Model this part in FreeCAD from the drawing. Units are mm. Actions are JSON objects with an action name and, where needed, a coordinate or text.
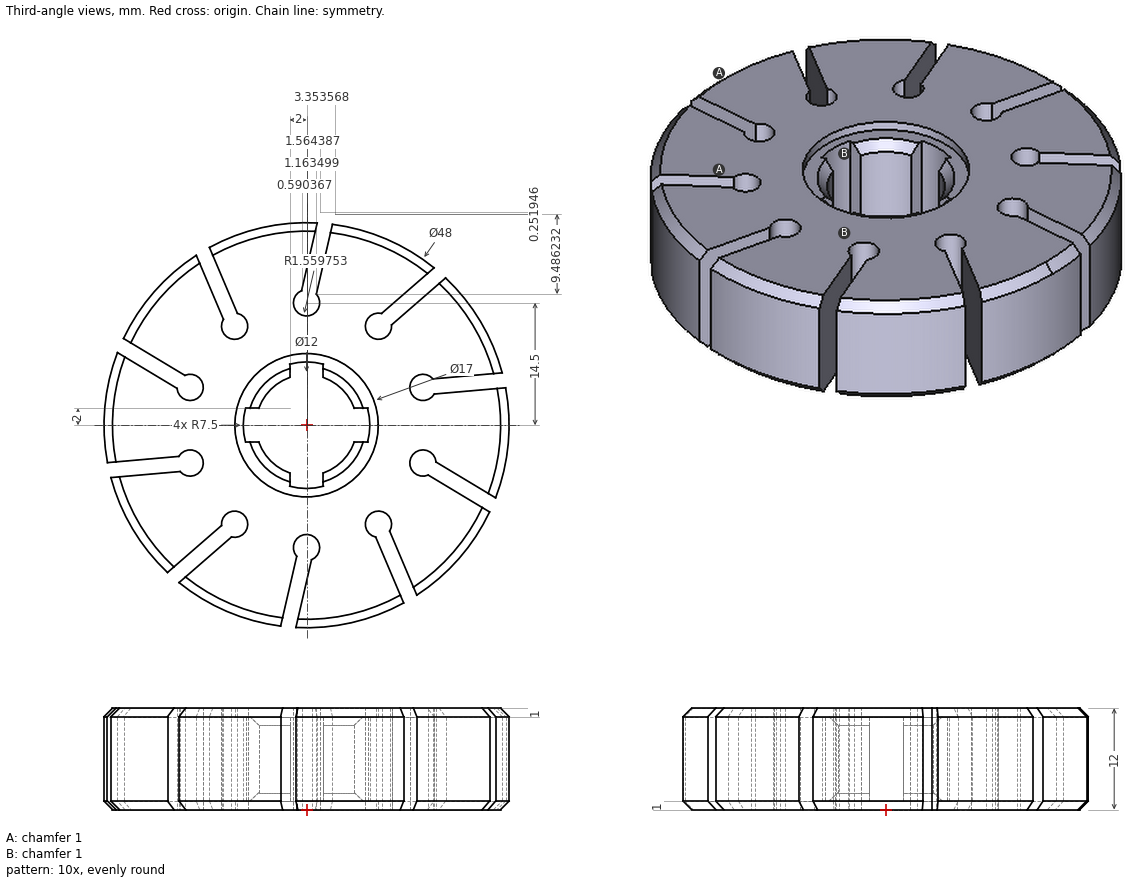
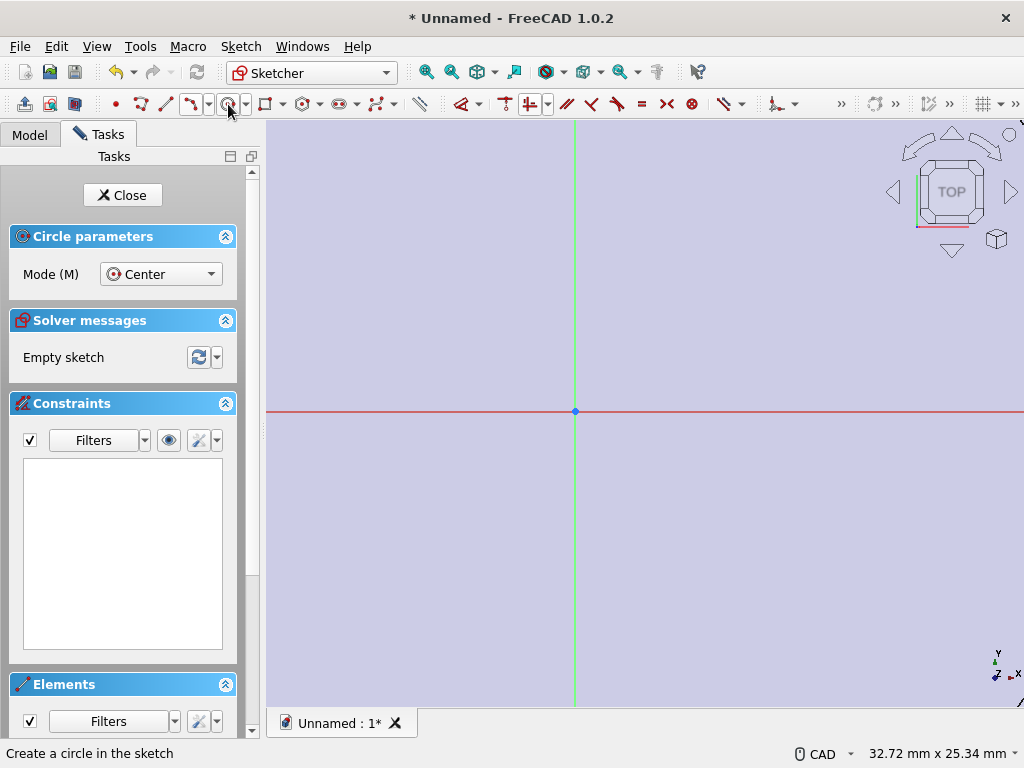
{"action": "left_click", "coordinate": [575, 412]}
{"action": "mouse_move", "coordinate": [715, 273]}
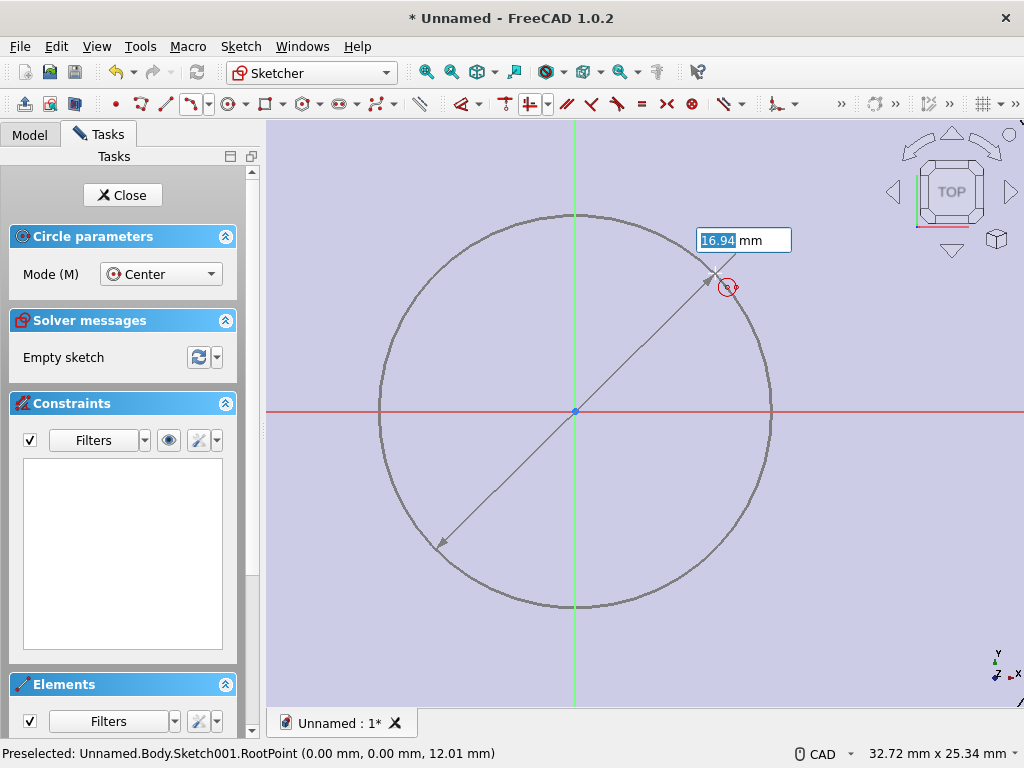
{"action": "type", "text": "17"}
{"action": "key", "text": "Return"}
{"action": "key", "text": "Escape"}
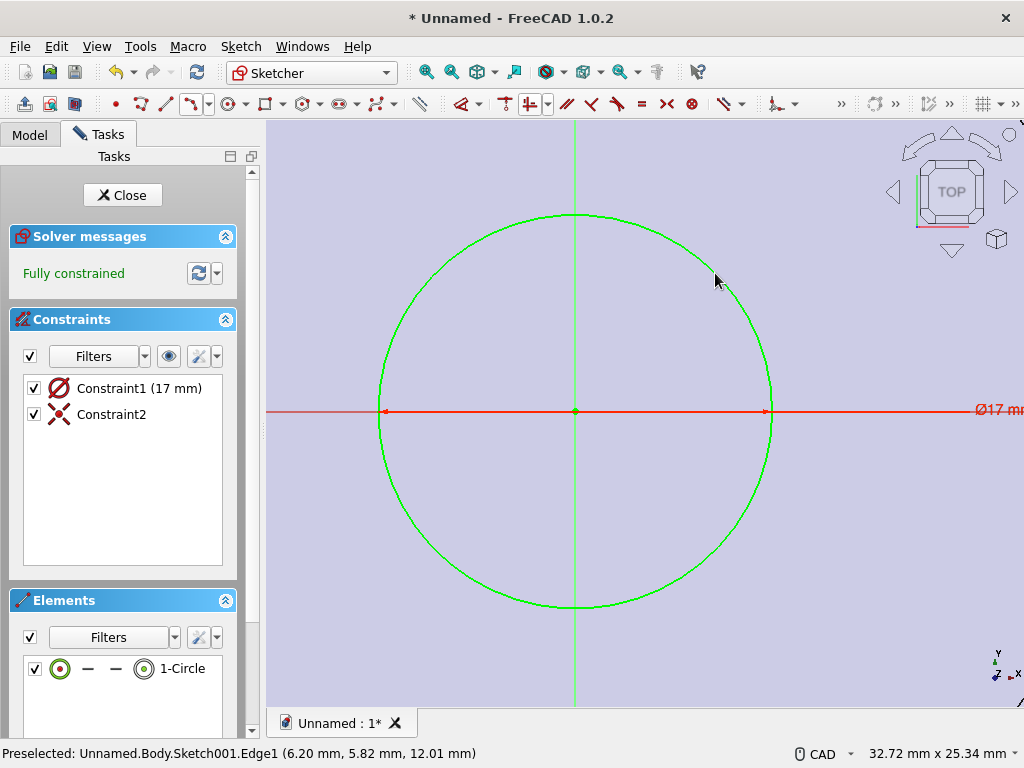
{"action": "left_click", "coordinate": [123, 195]}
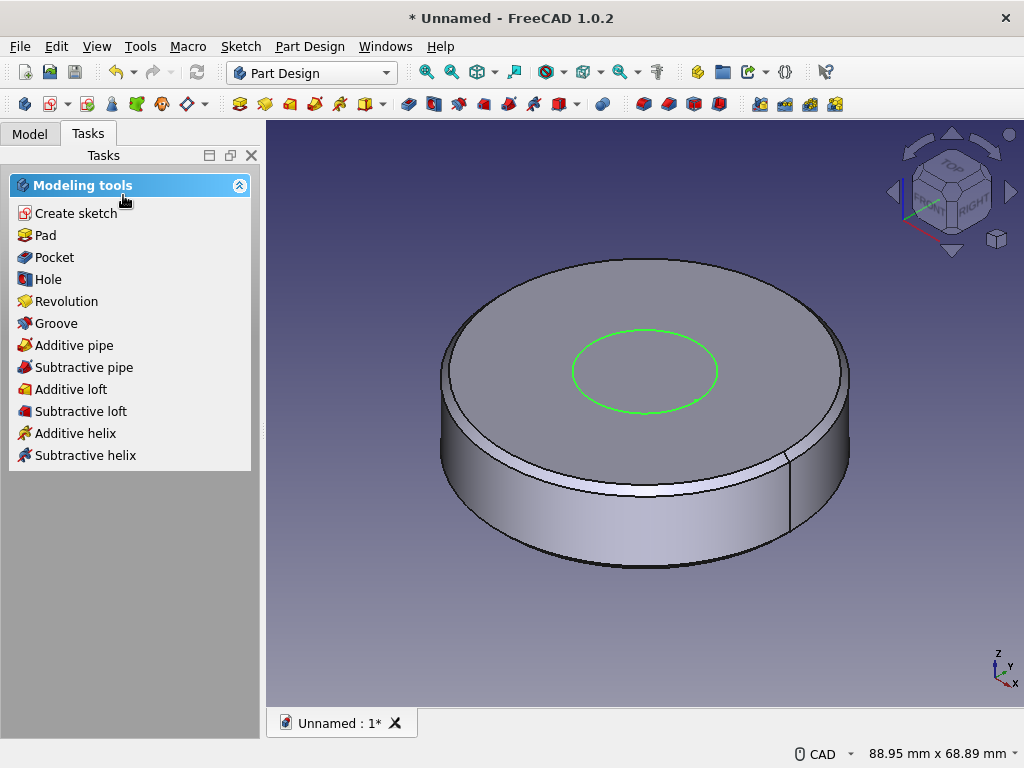
{"action": "left_click", "coordinate": [409, 104]}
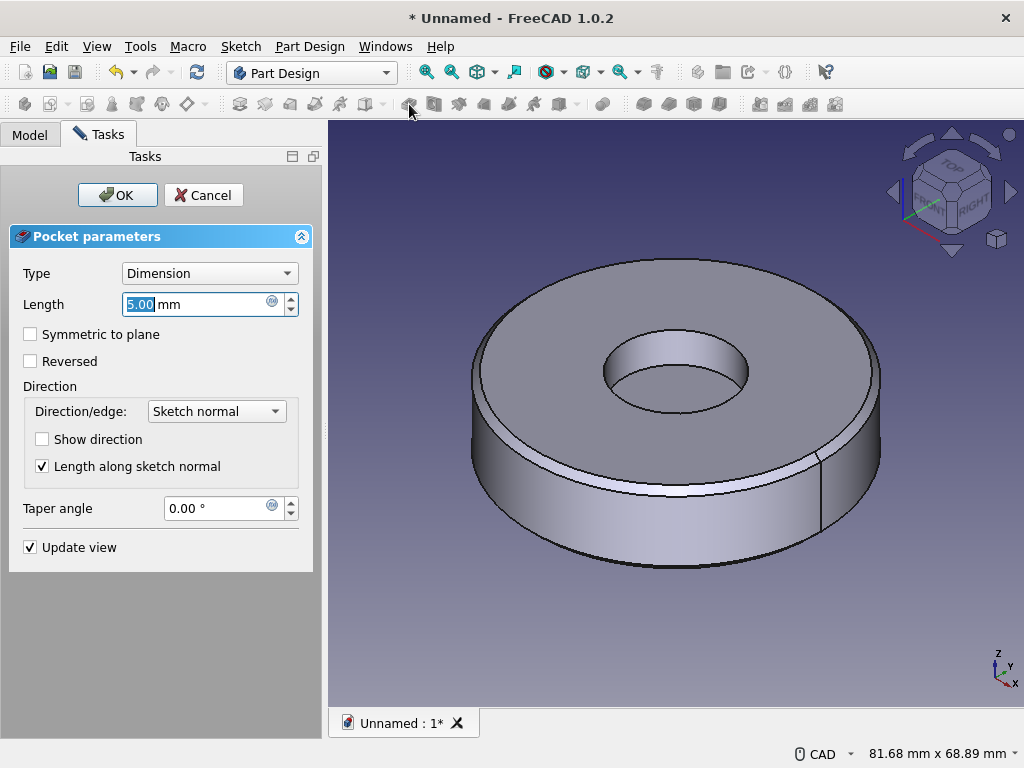
{"action": "type", "text": "1"}
{"action": "key", "text": "Tab"}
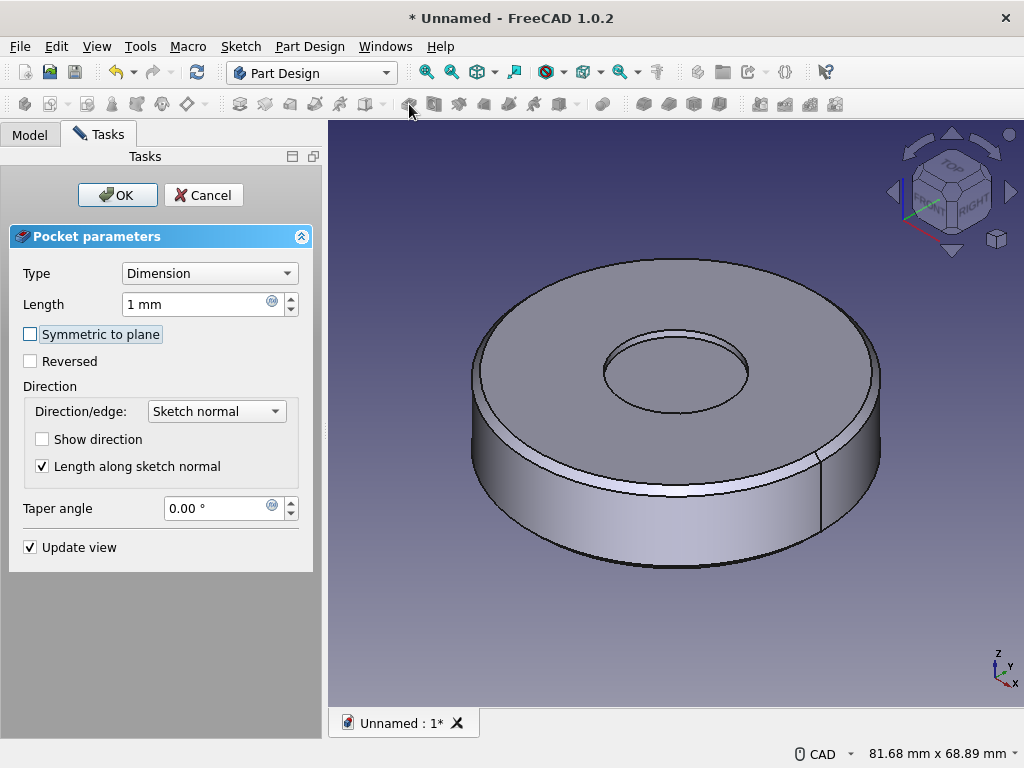
{"action": "left_click", "coordinate": [118, 195]}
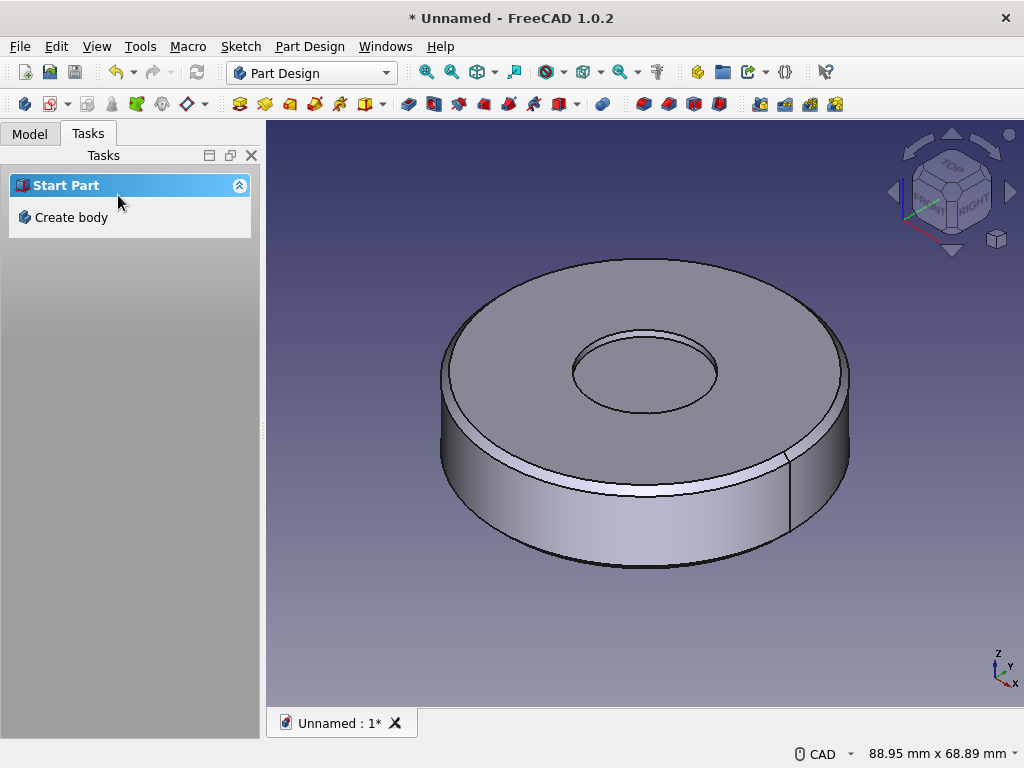
{"action": "left_click", "coordinate": [30, 134]}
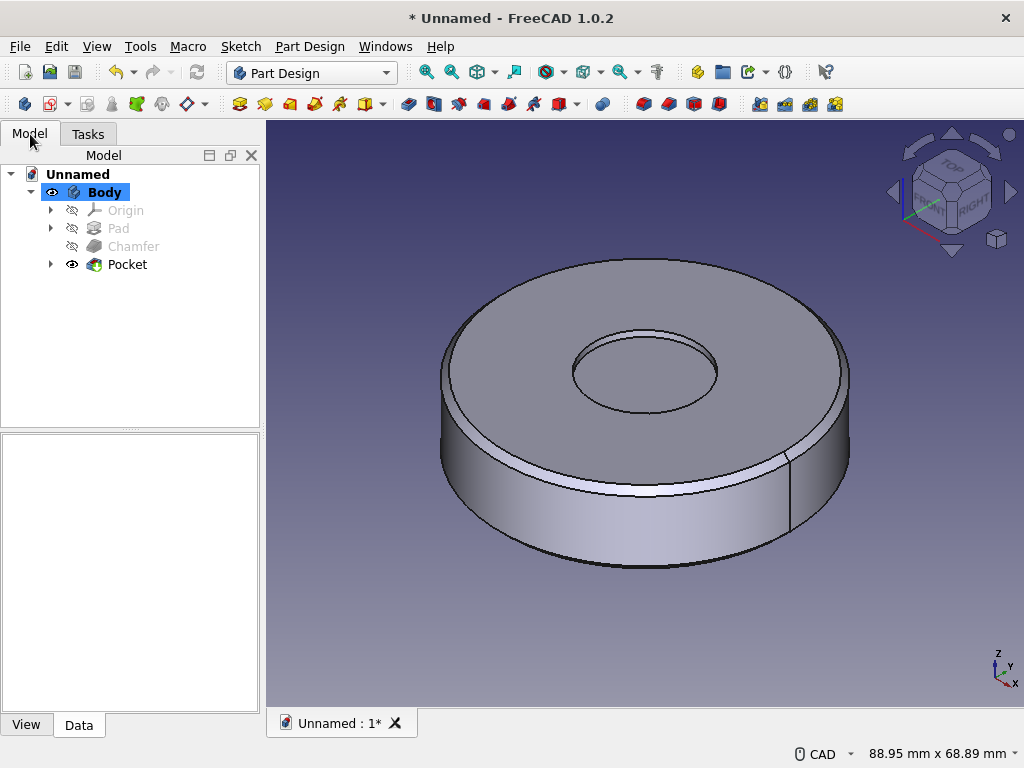
{"action": "left_click", "coordinate": [51, 210]}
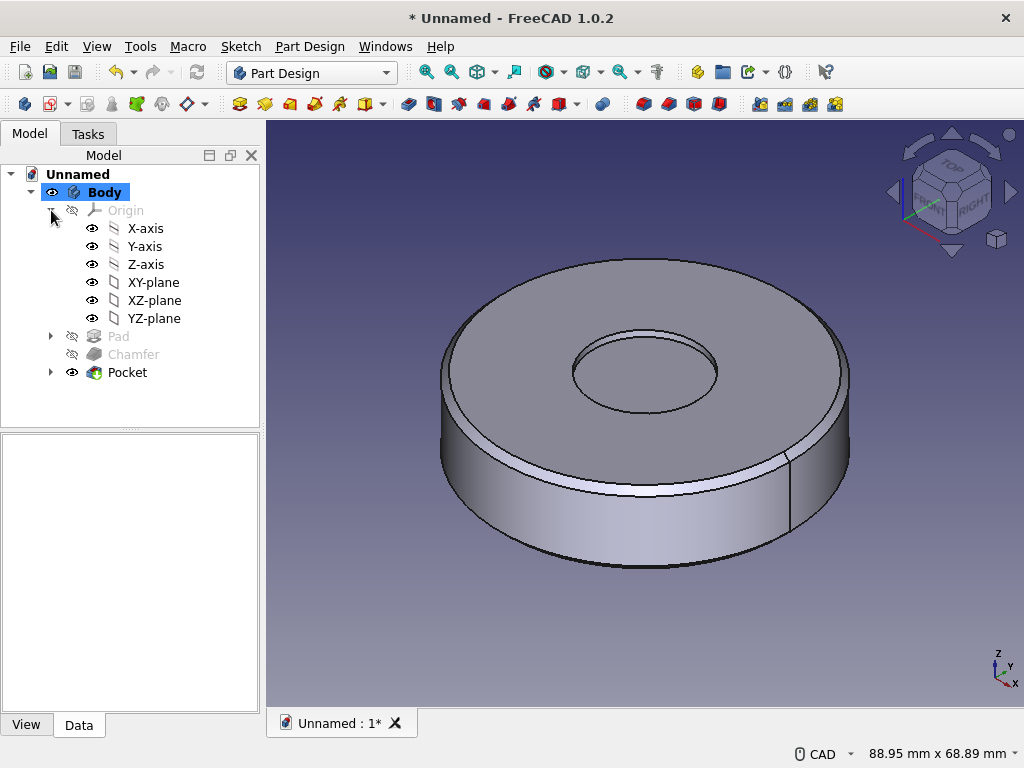
{"action": "left_click", "coordinate": [137, 282]}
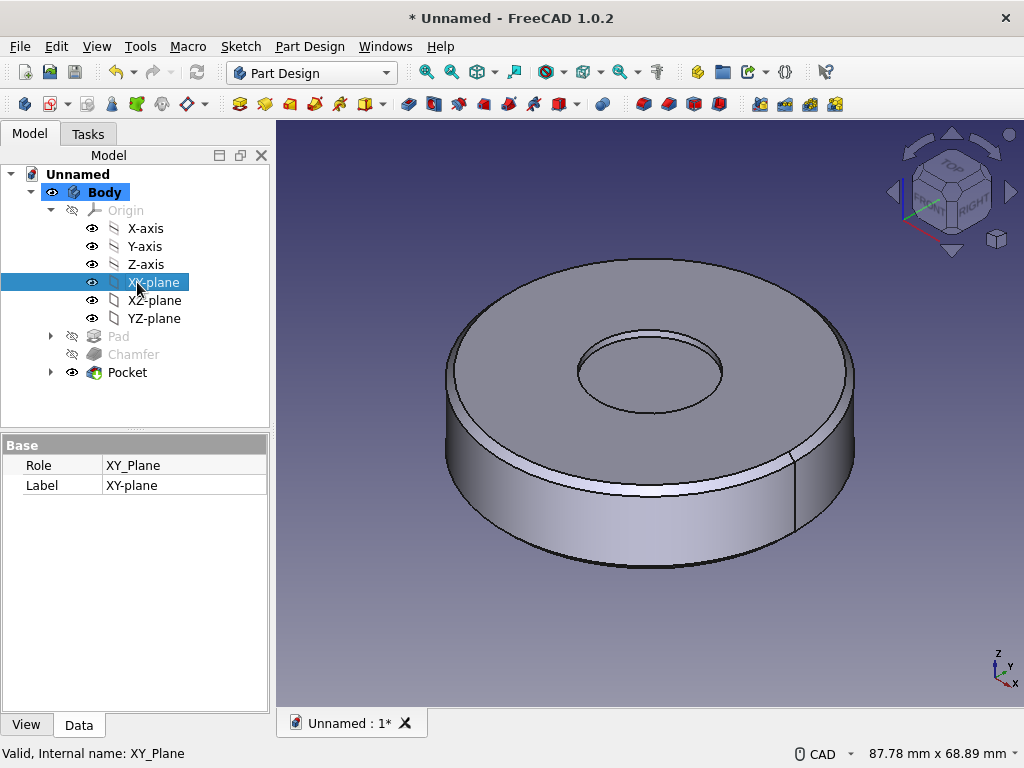
{"action": "left_click", "coordinate": [186, 104]}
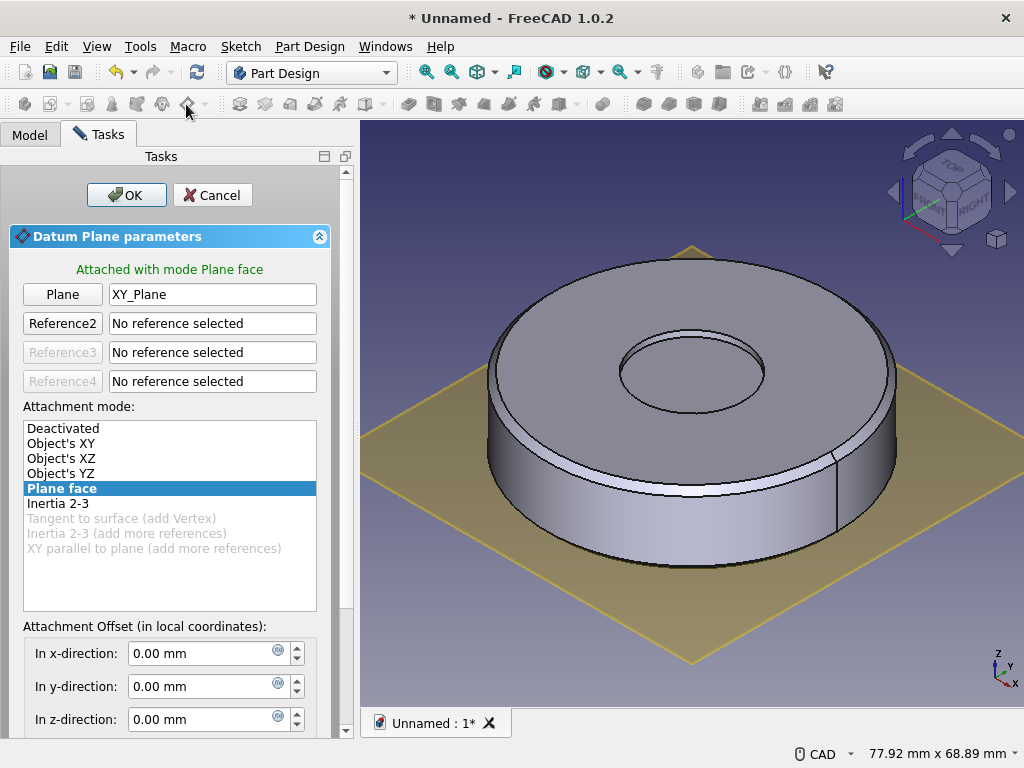
{"action": "triple_click", "coordinate": [210, 720]}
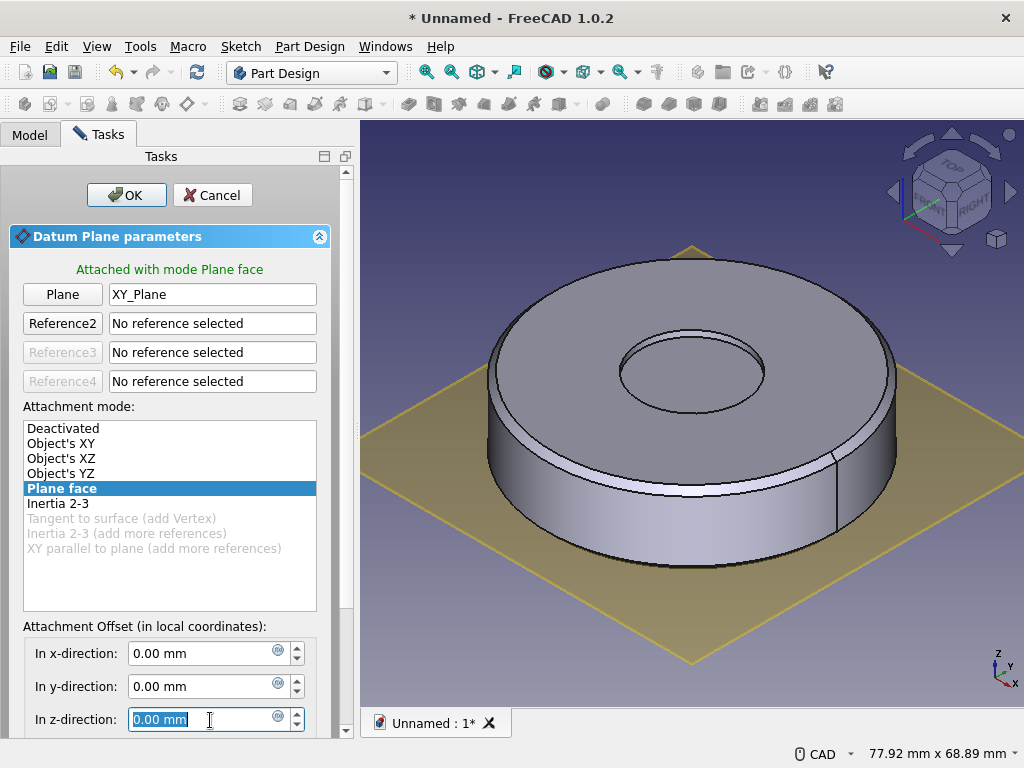
{"action": "type", "text": "1"}
{"action": "key", "text": "Tab"}